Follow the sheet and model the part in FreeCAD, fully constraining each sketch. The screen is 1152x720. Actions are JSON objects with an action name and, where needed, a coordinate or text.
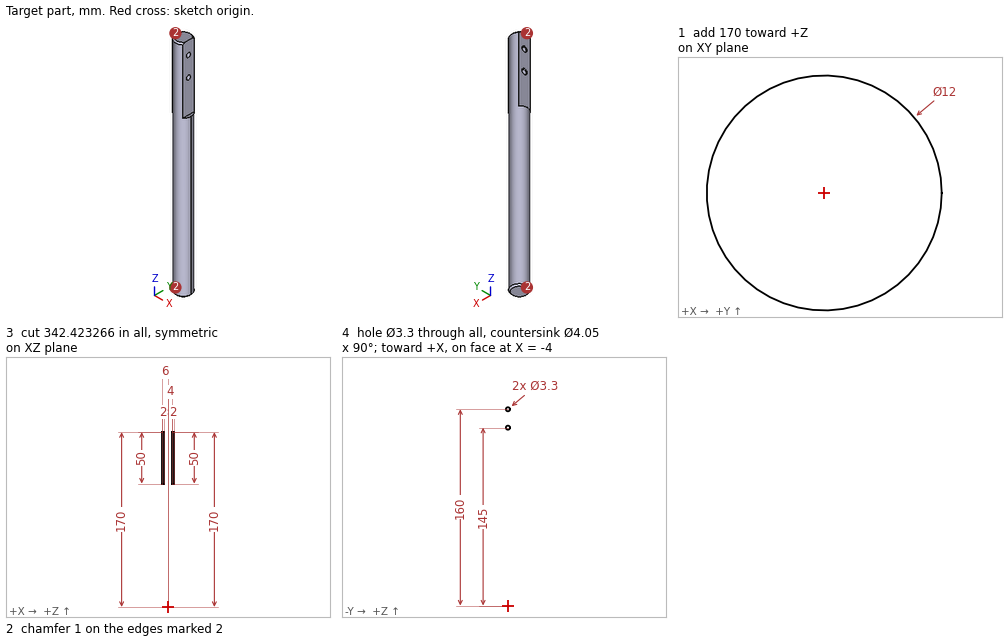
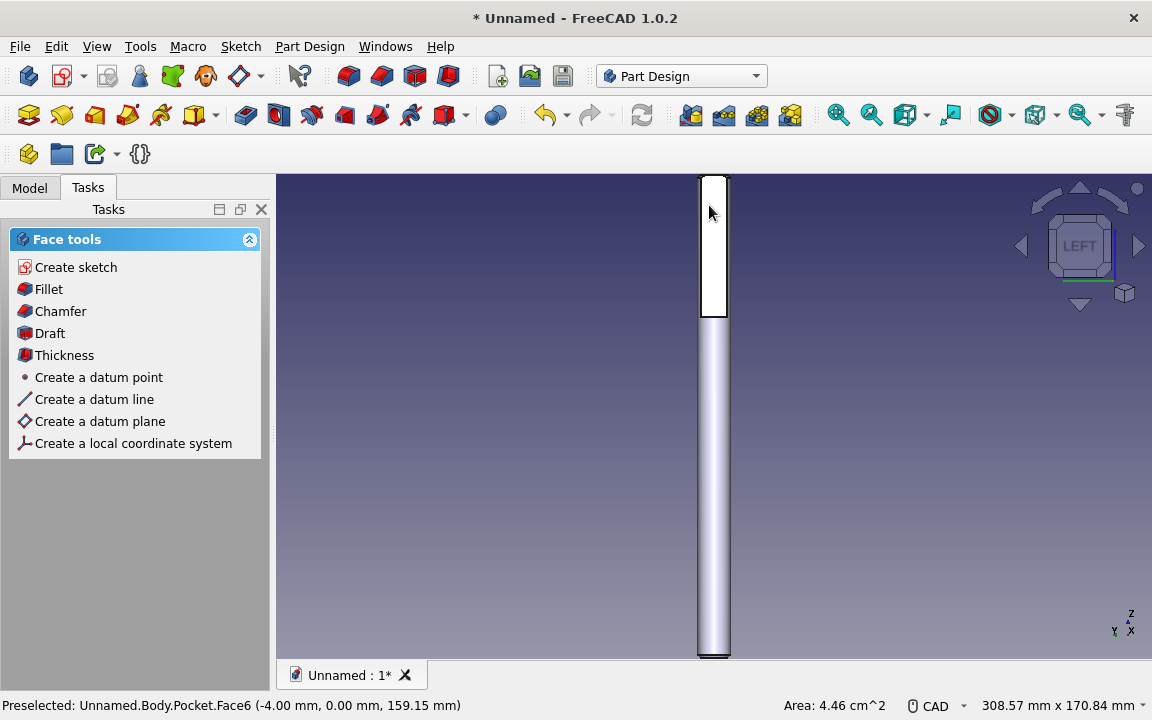
{"action": "left_click", "coordinate": [62, 76]}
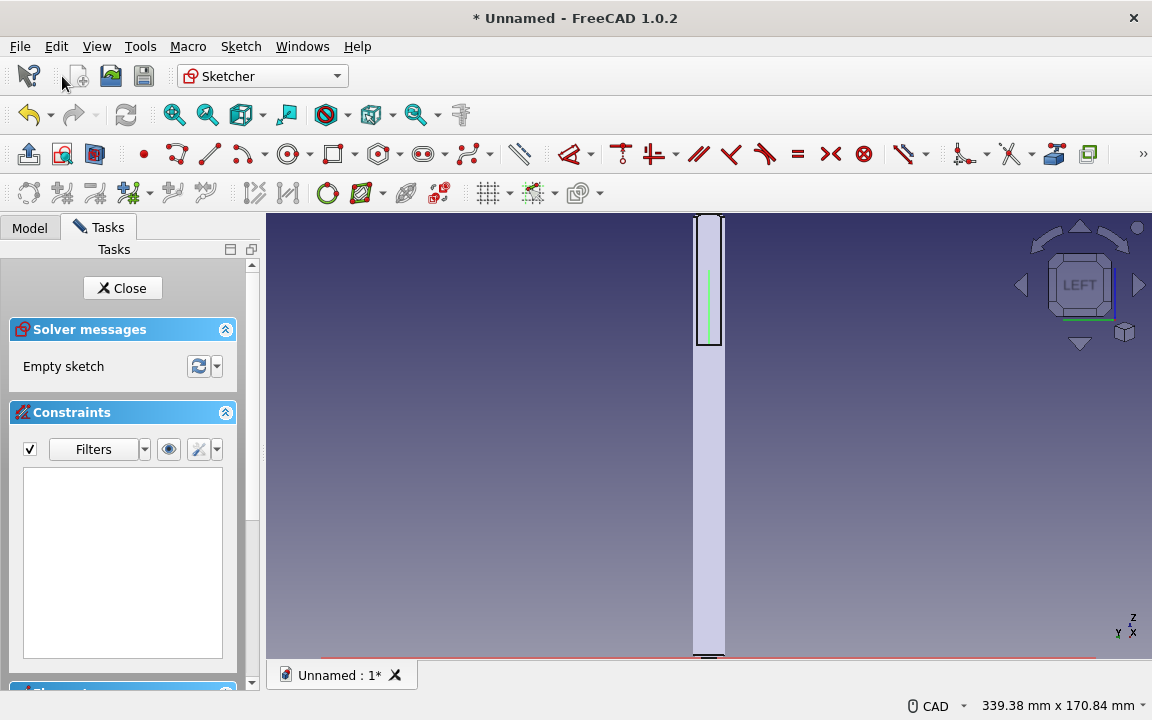
{"action": "key", "text": "q s"}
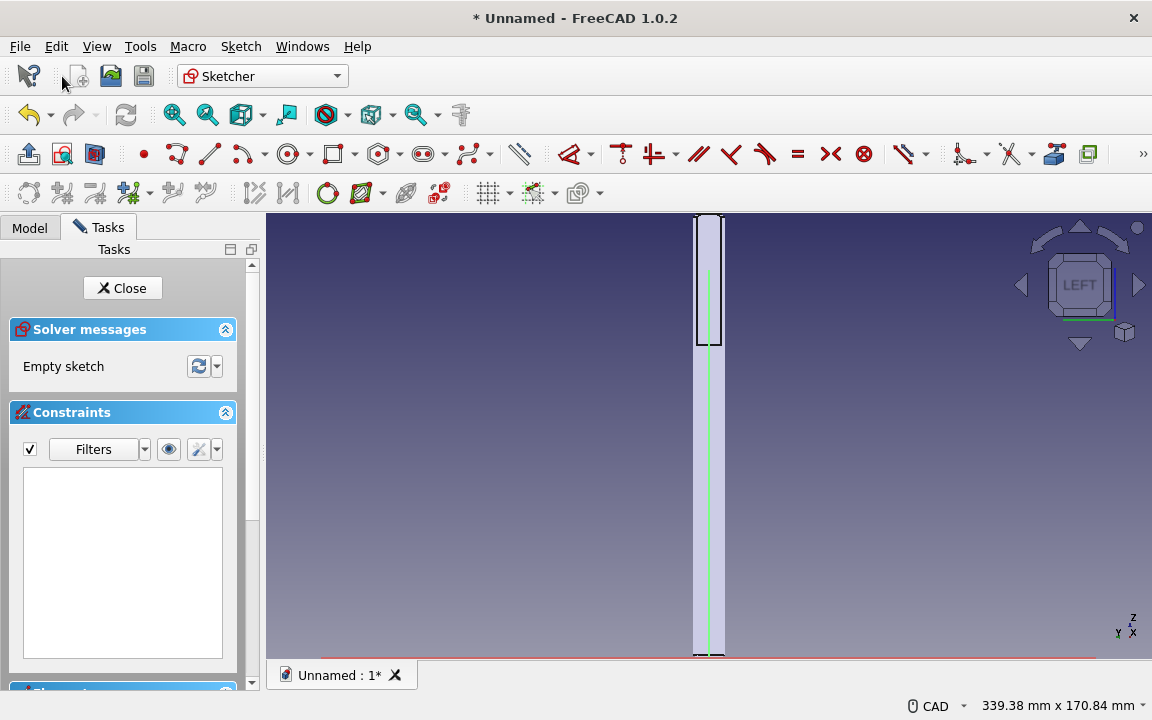
{"action": "scroll", "coordinate": [640, 436], "scroll_direction": "down", "scroll_amount": 5}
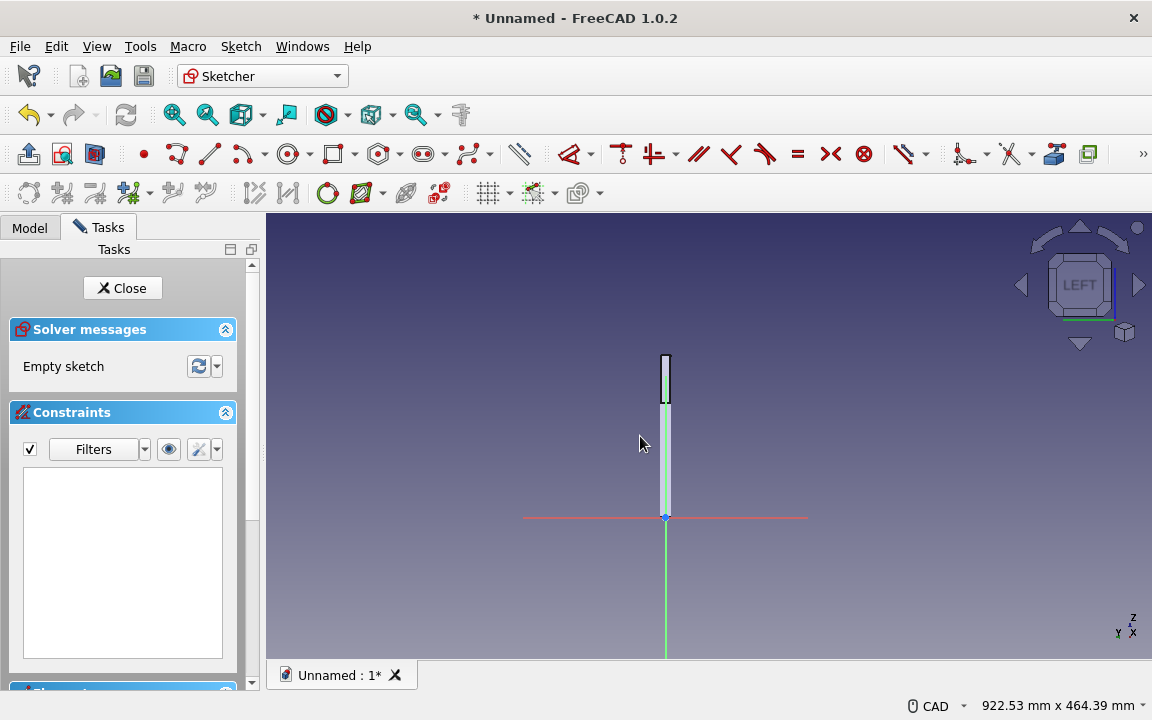
{"action": "scroll", "coordinate": [667, 367], "scroll_direction": "up", "scroll_amount": 14}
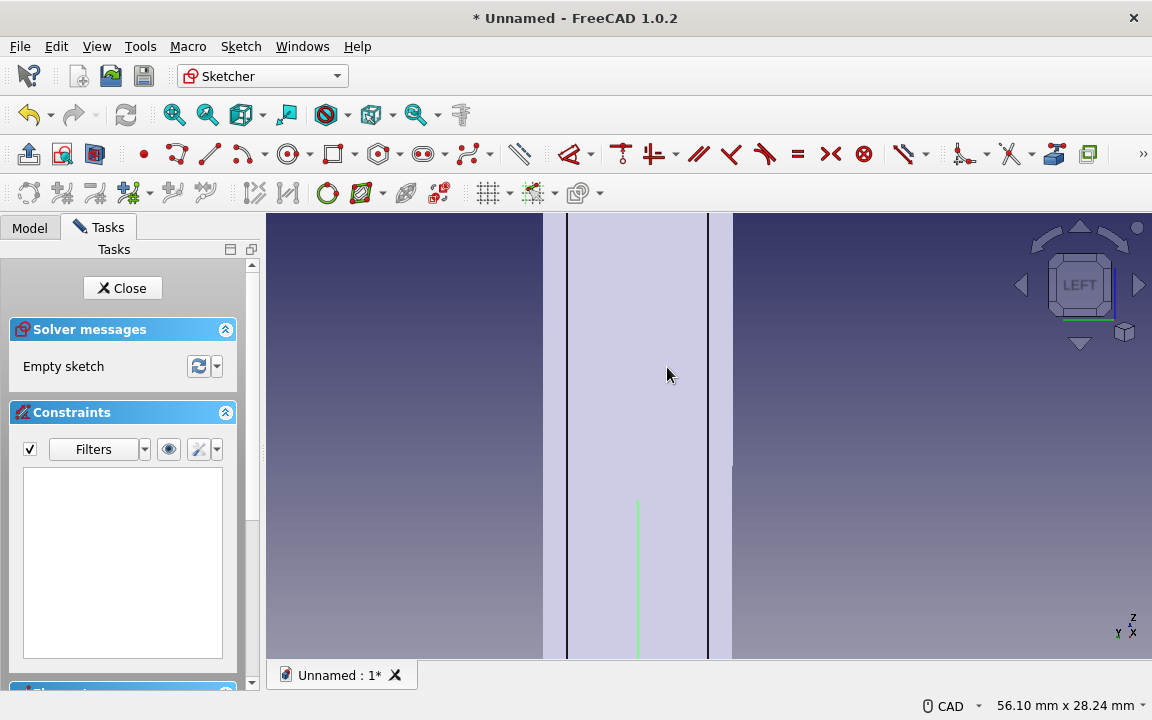
{"action": "key", "text": "g c"}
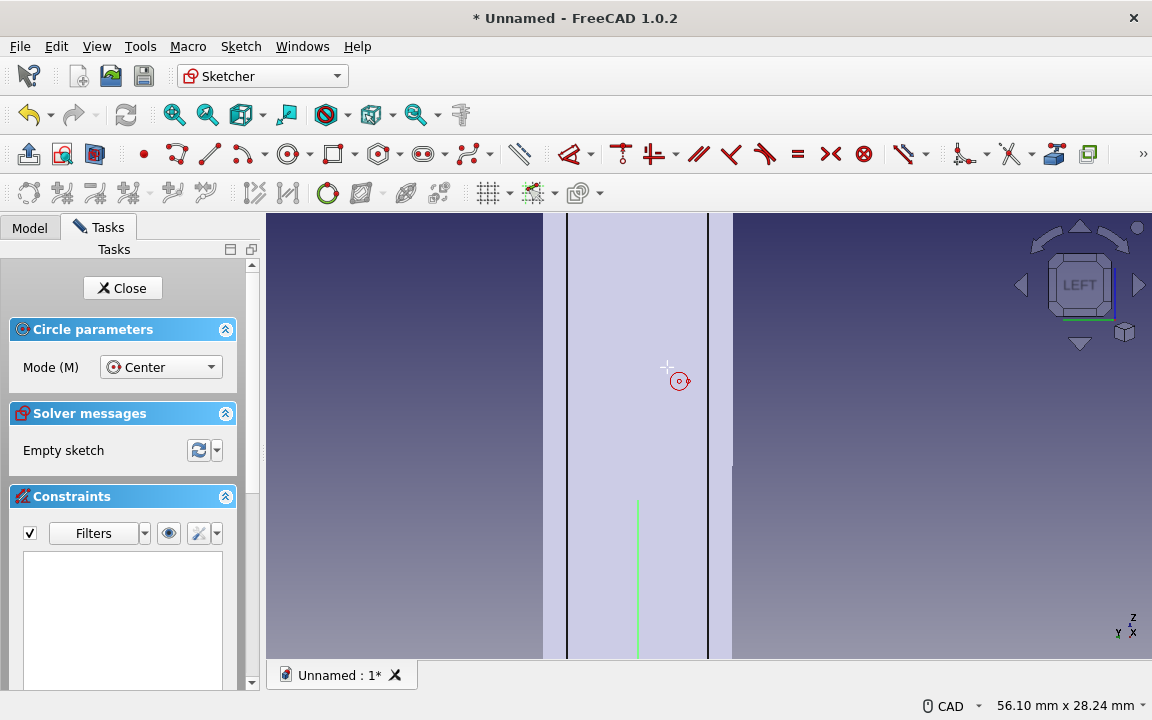
{"action": "left_click", "coordinate": [638, 317]}
{"action": "mouse_move", "coordinate": [656, 299]}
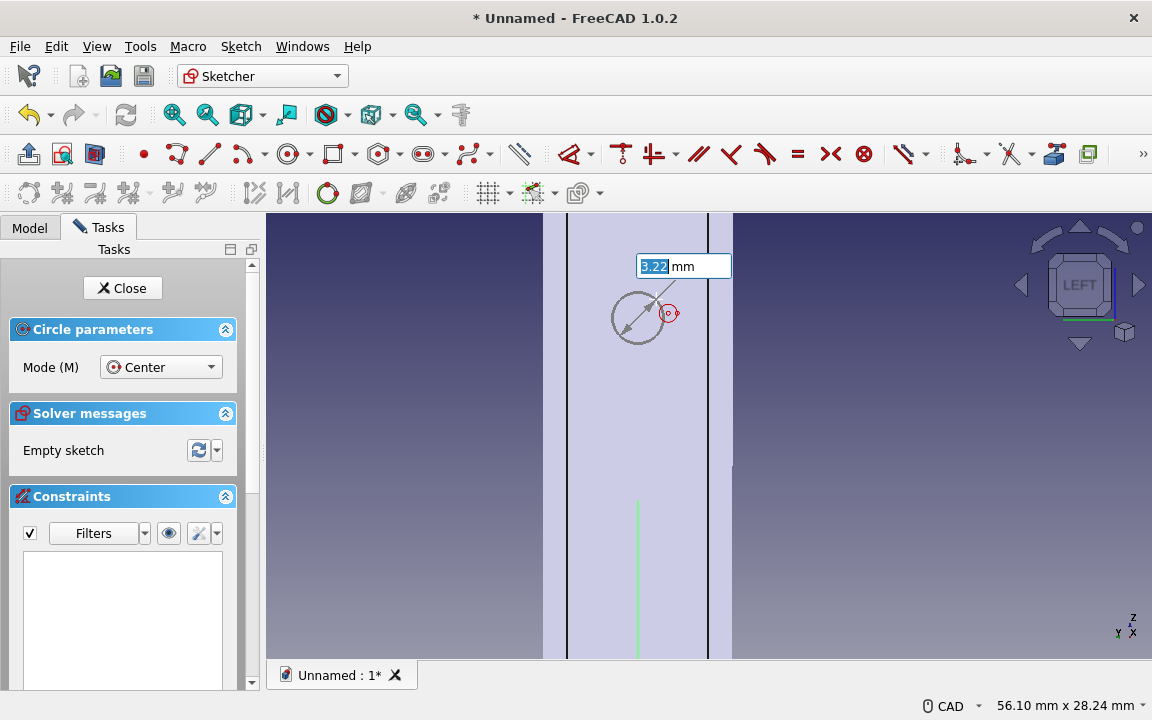
{"action": "type", "text": "3.3"}
{"action": "key", "text": "Return"}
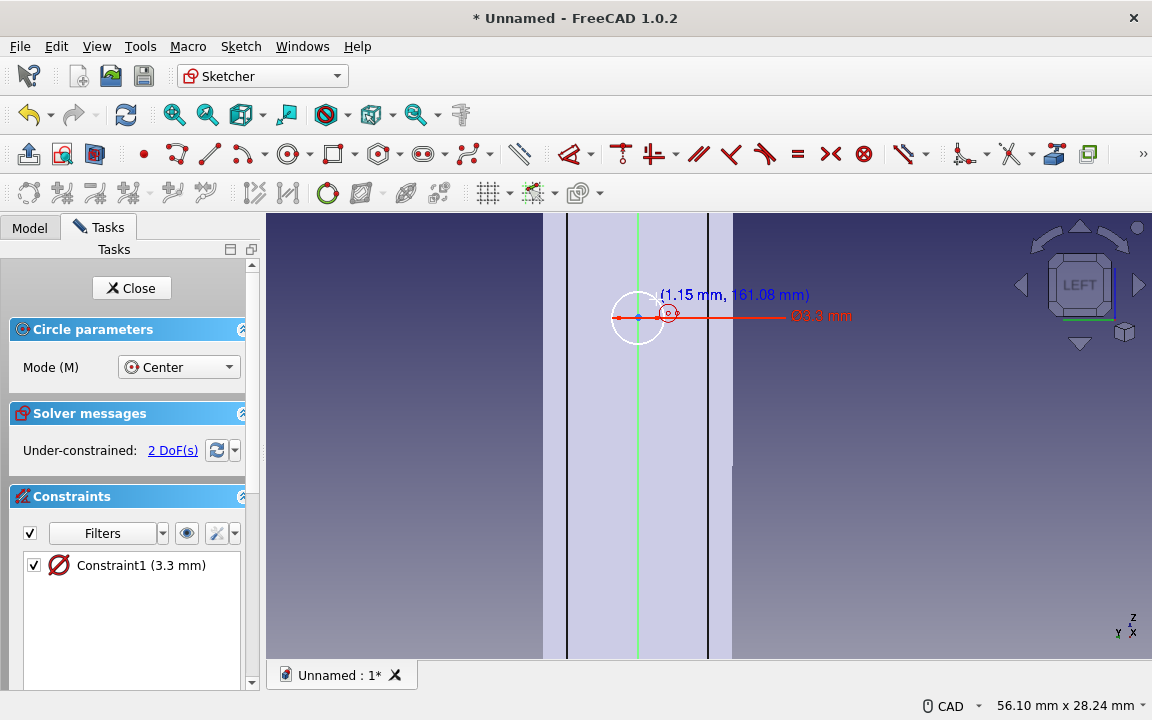
{"action": "left_click", "coordinate": [638, 554]}
{"action": "mouse_move", "coordinate": [656, 536]}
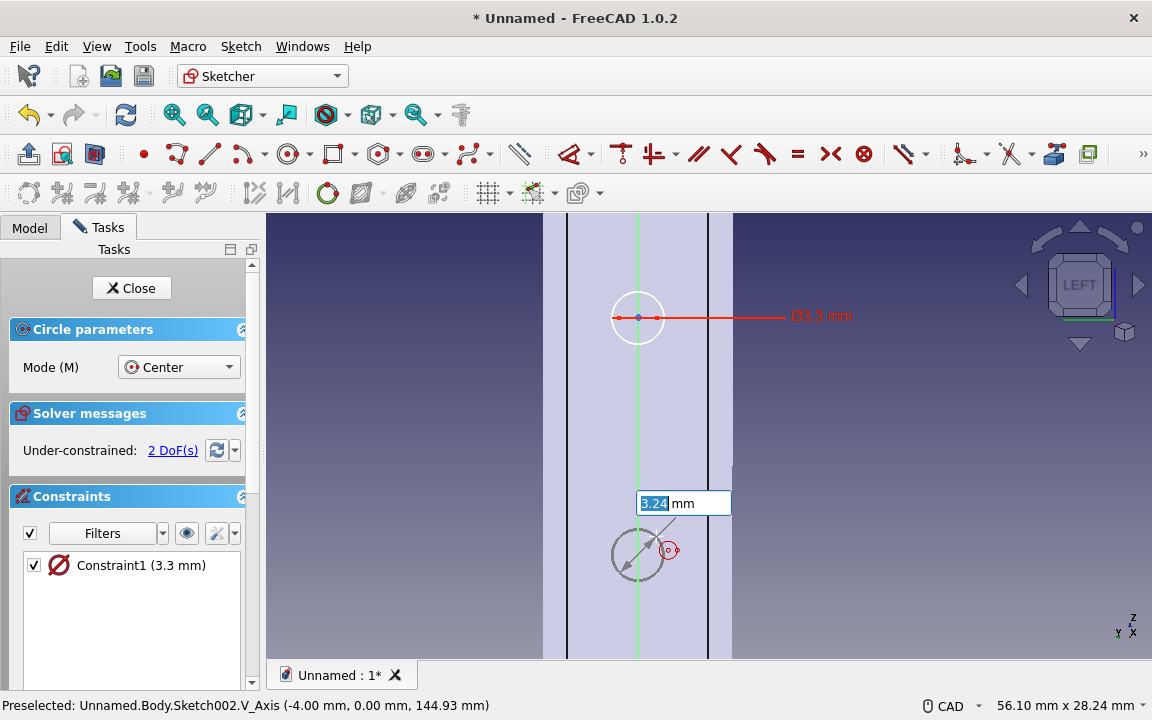
{"action": "type", "text": "3.3"}
{"action": "key", "text": "Return"}
{"action": "key", "text": "Escape"}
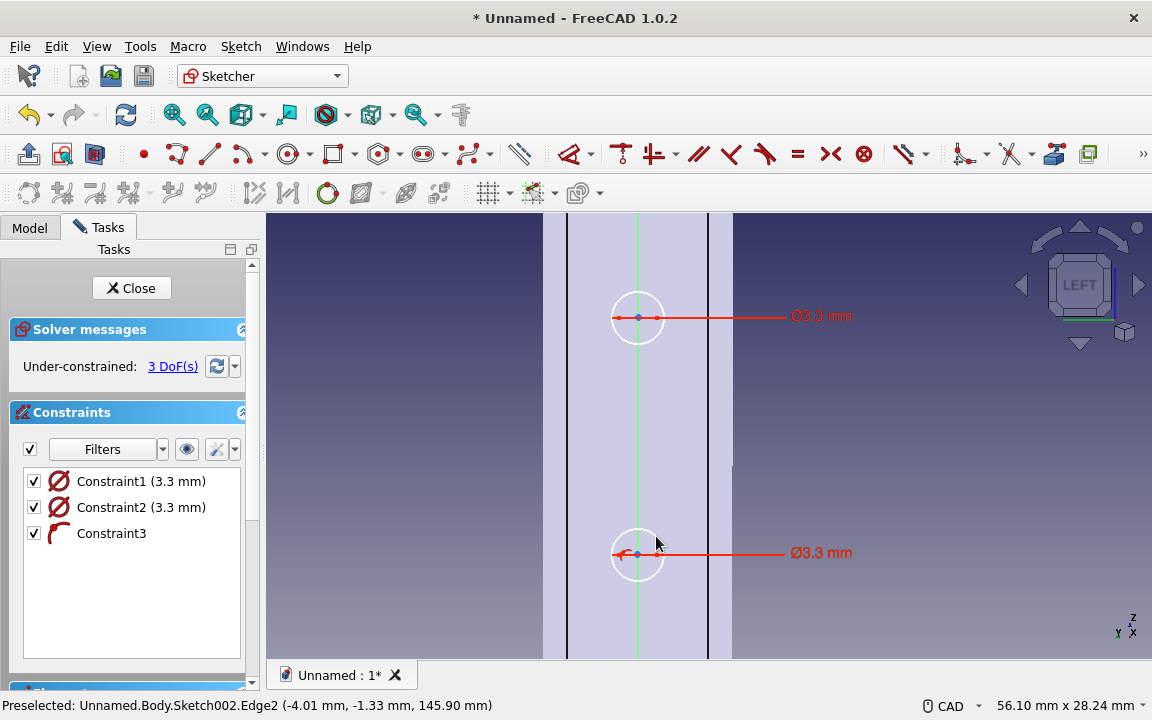
{"action": "left_click", "coordinate": [638, 318]}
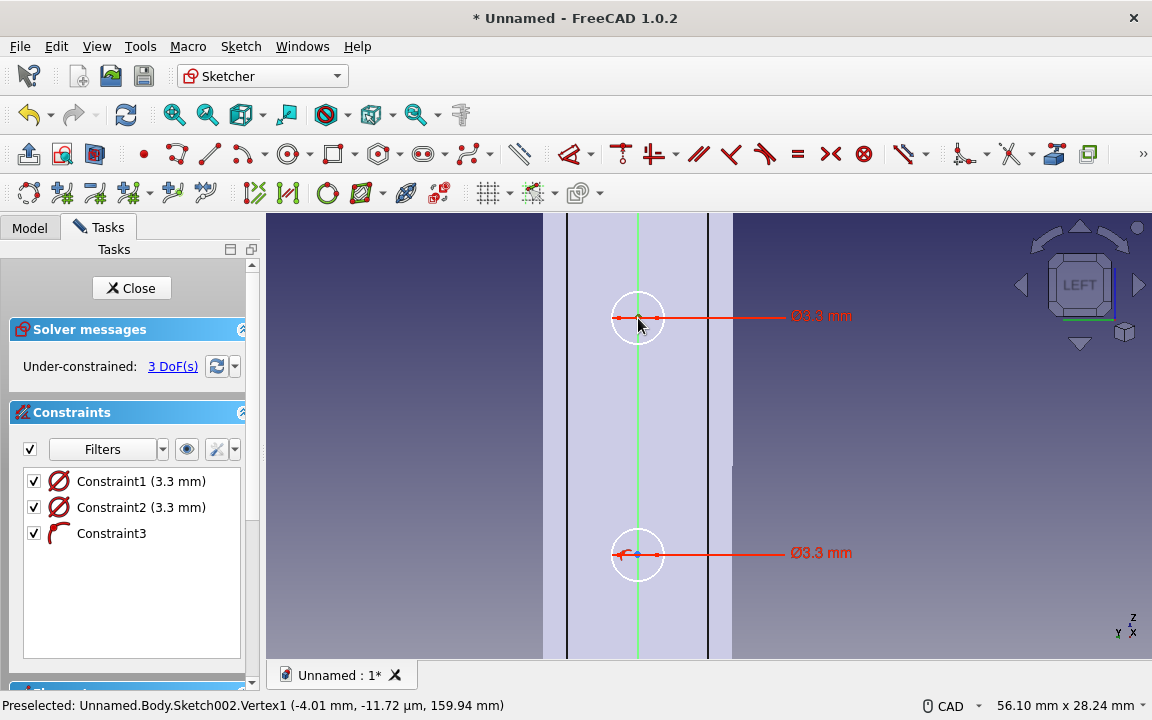
{"action": "left_click", "coordinate": [638, 492]}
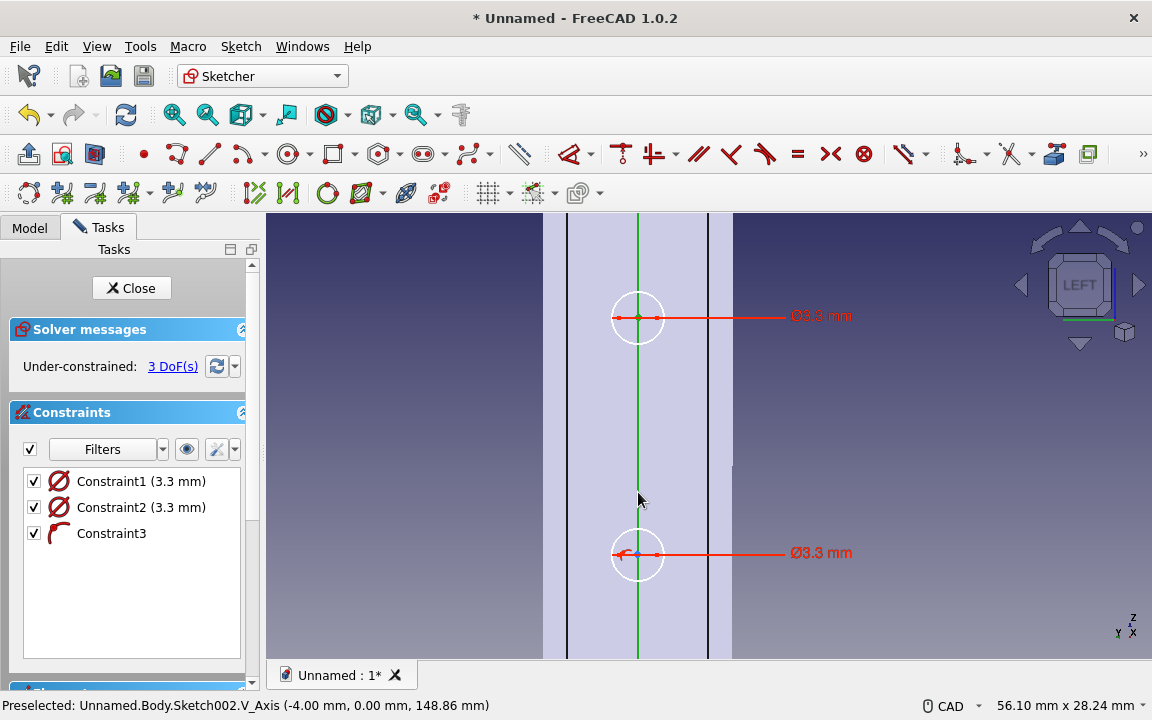
{"action": "key", "text": "c"}